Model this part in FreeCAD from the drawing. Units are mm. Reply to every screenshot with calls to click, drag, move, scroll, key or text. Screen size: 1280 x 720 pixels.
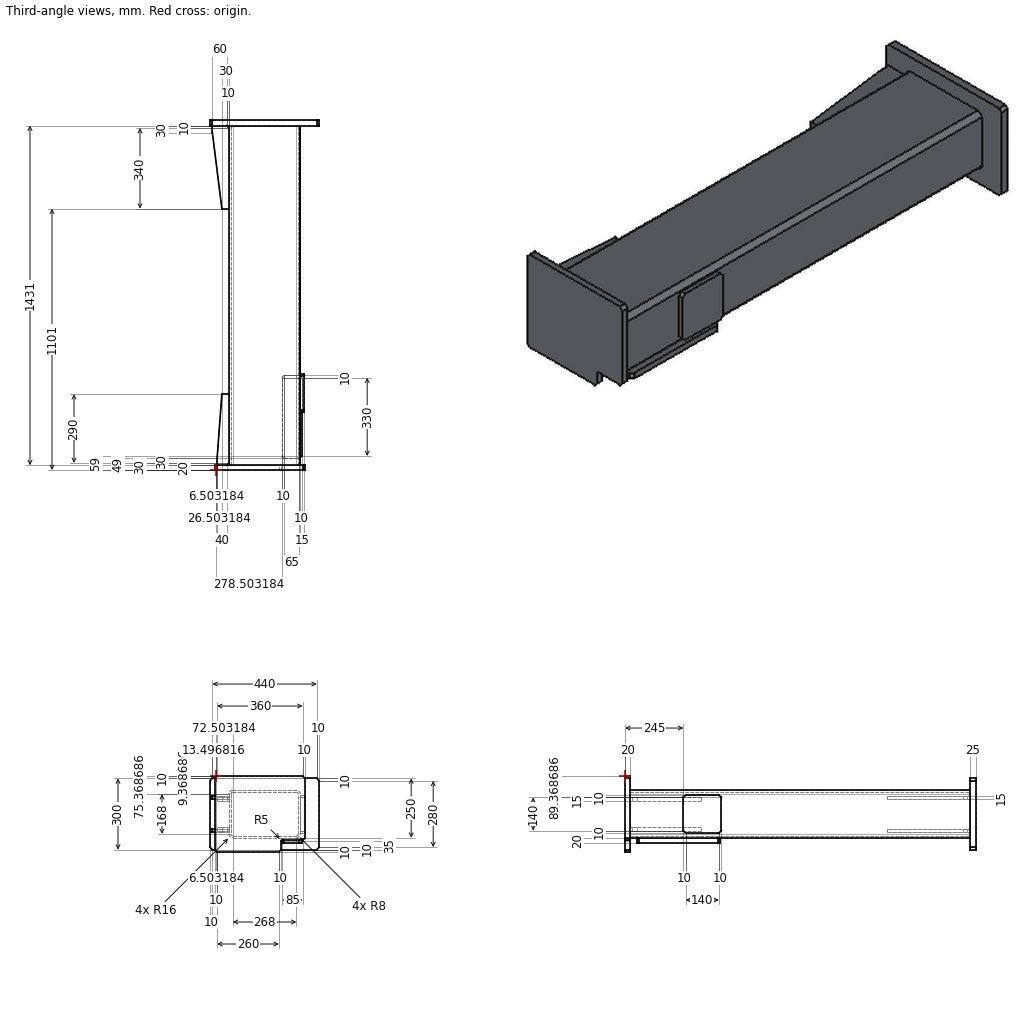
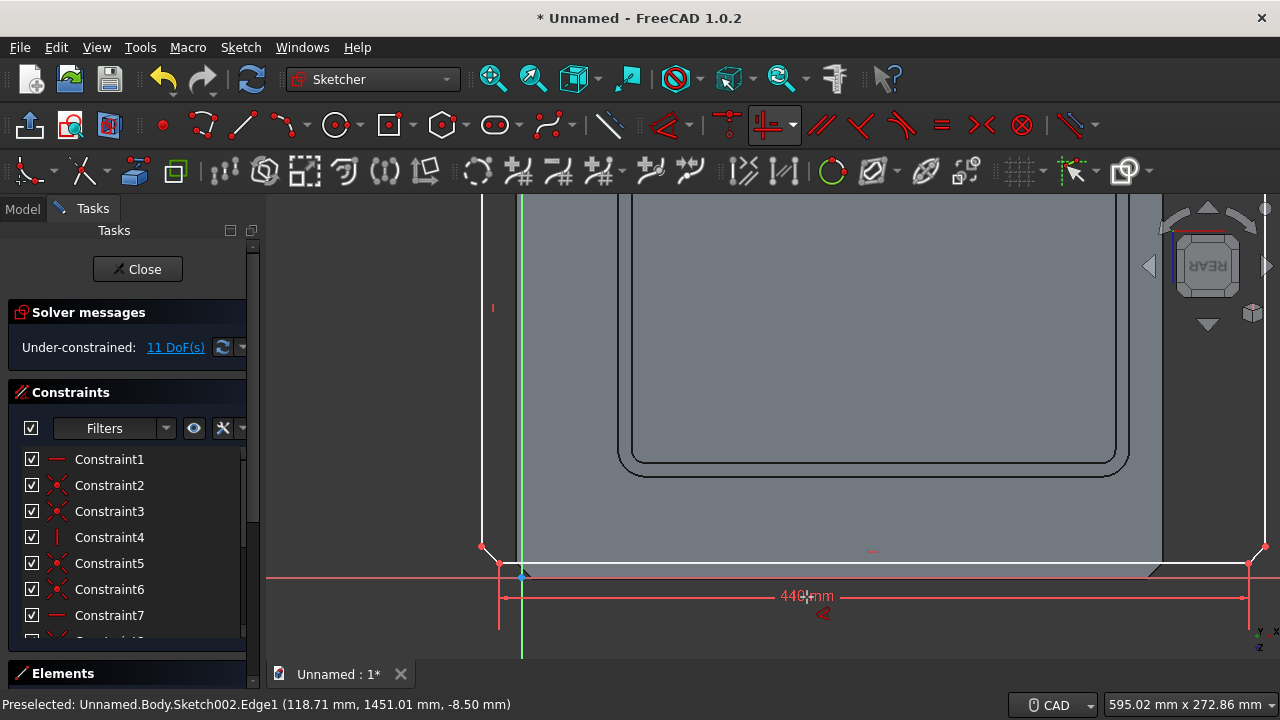
scroll(499, 563, down, 3)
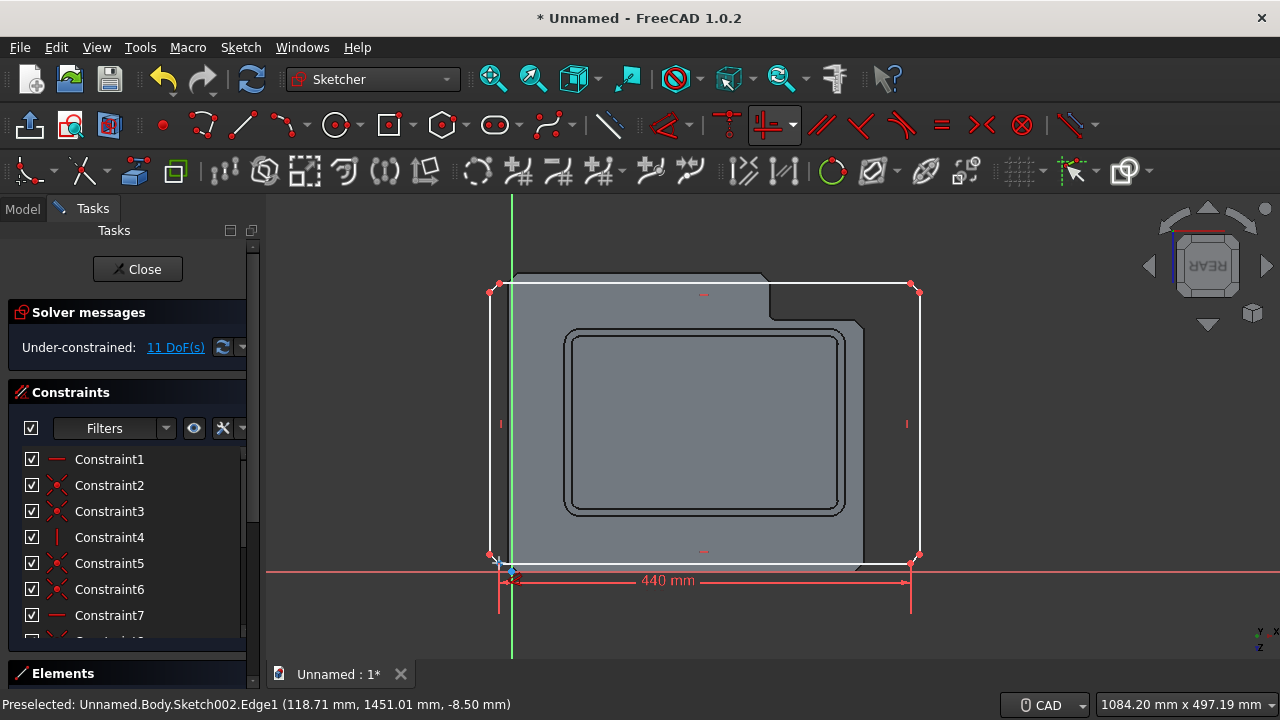
click(920, 476)
click(954, 423)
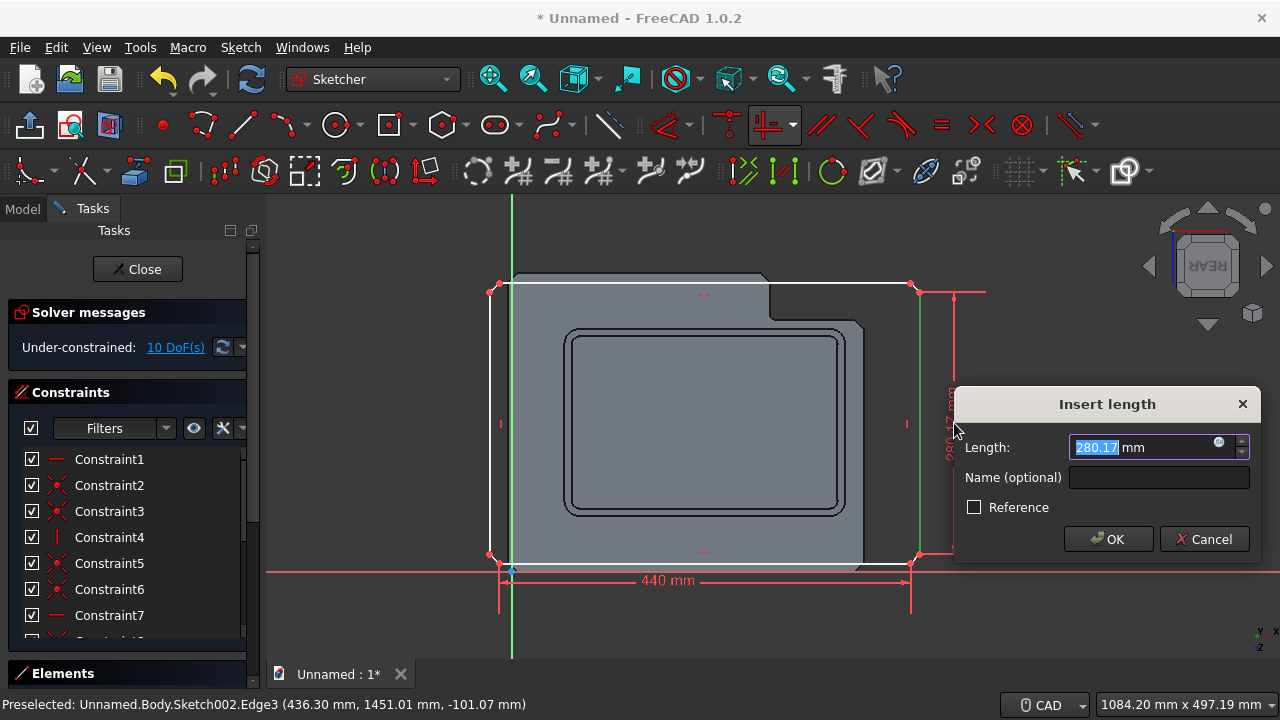
text(280)
key(Return)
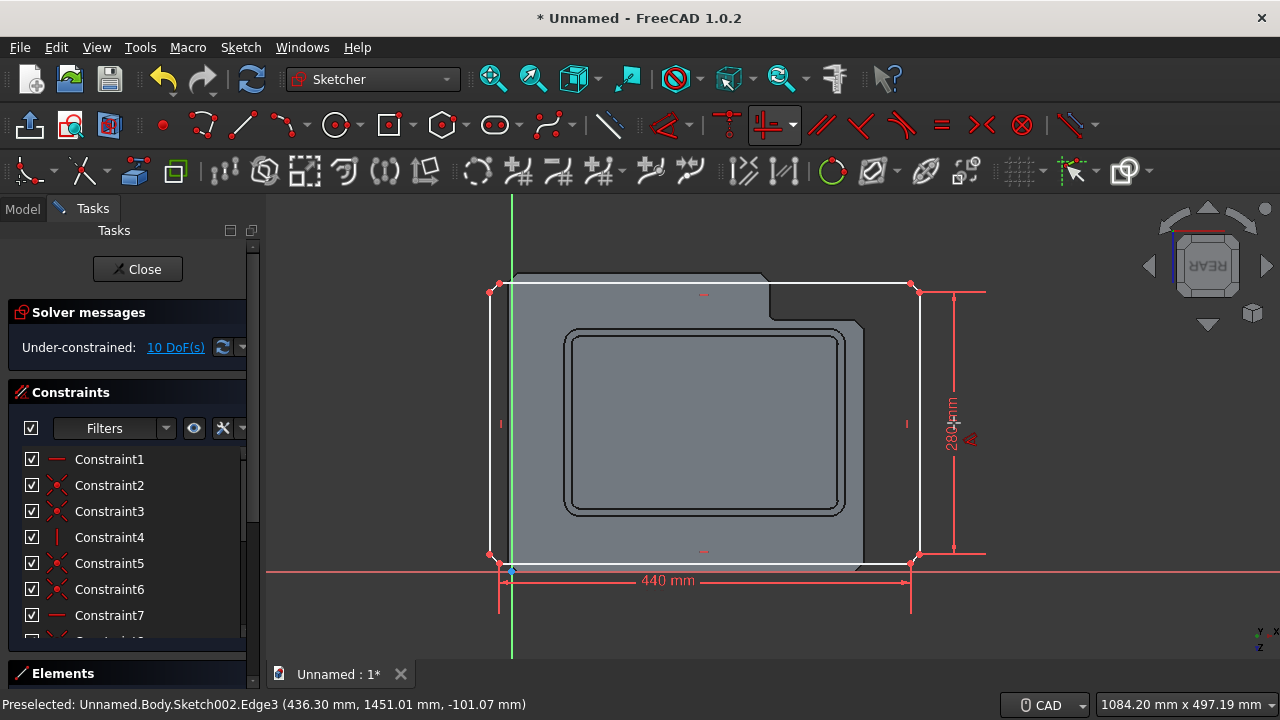
click(787, 283)
click(705, 249)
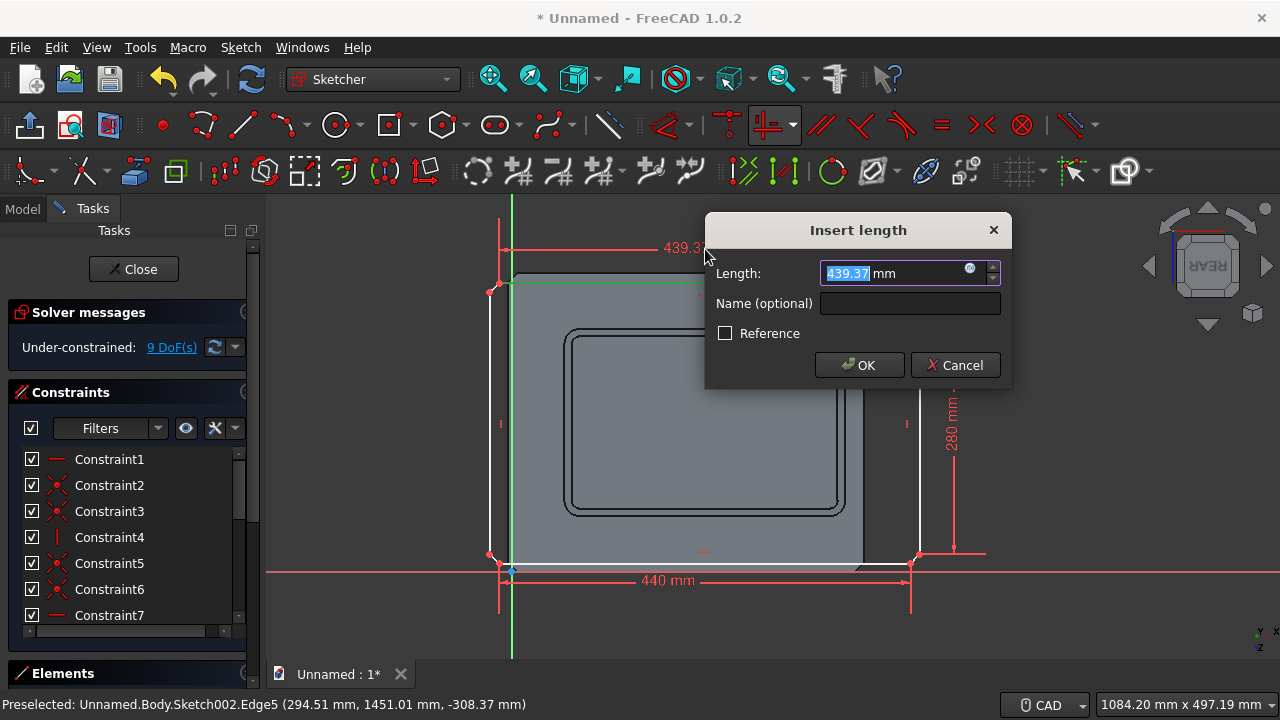
text(440)
key(Return)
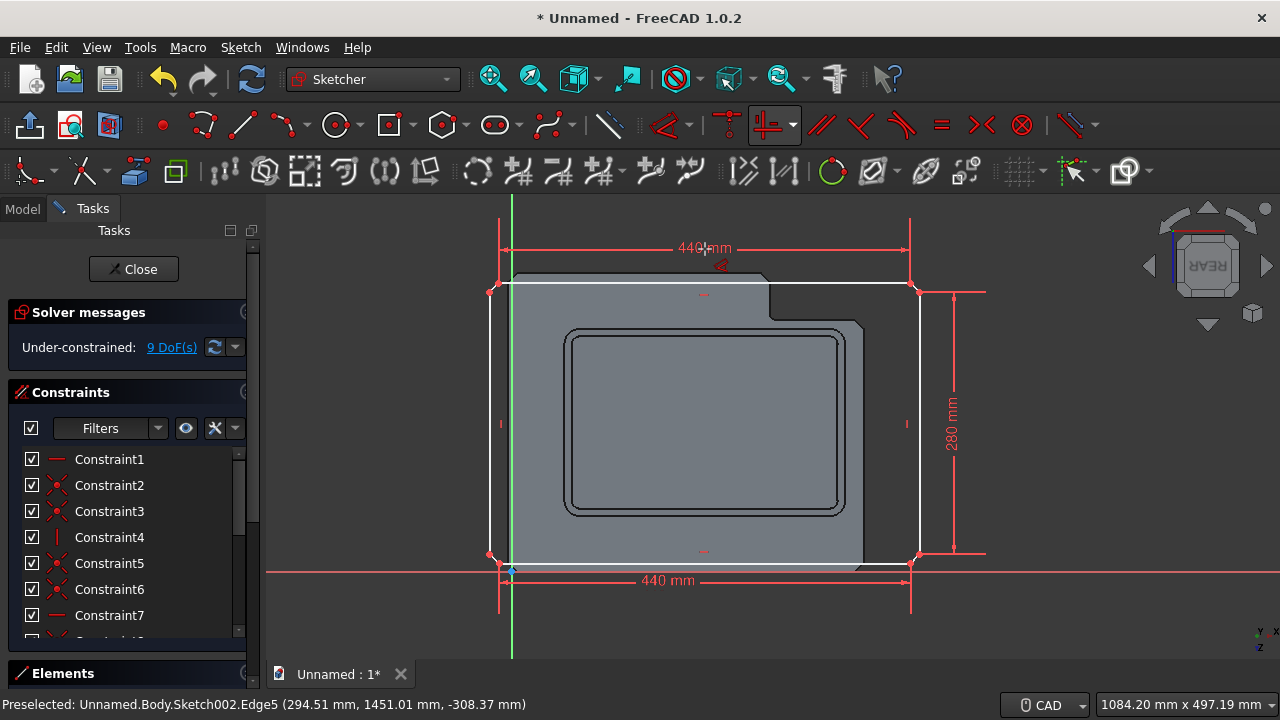
click(490, 371)
click(456, 423)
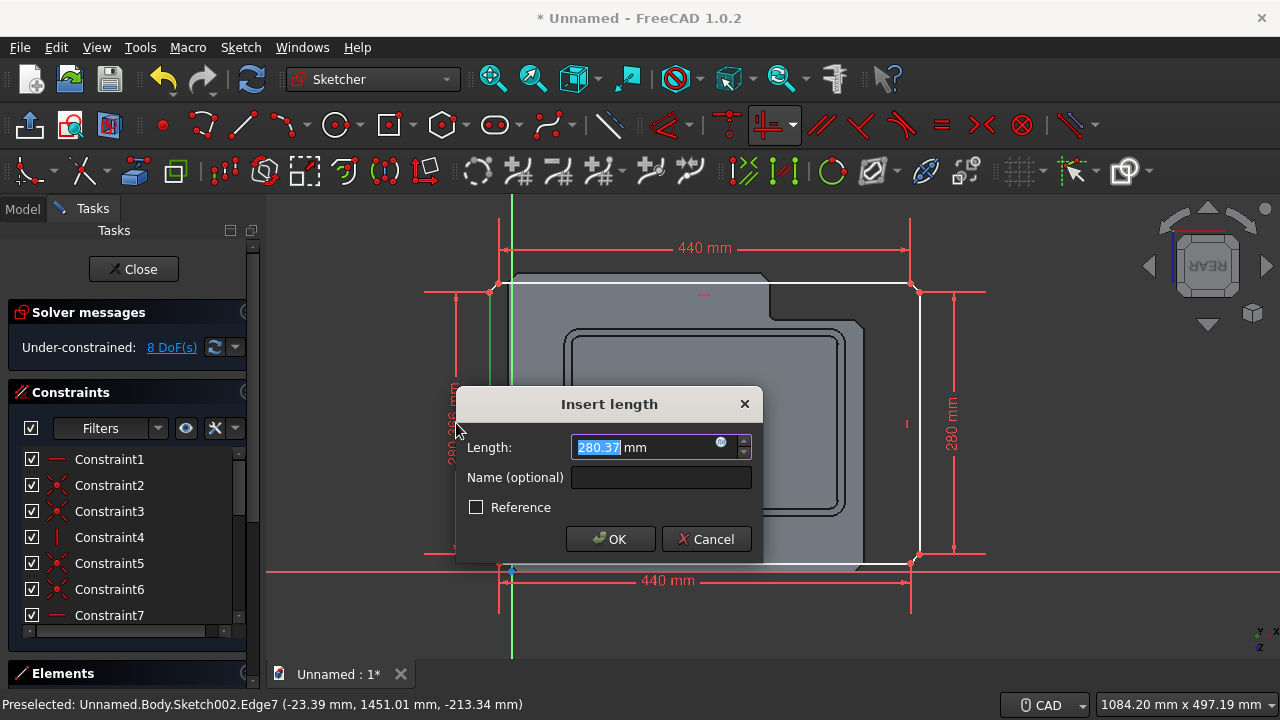
text(280)
key(Return)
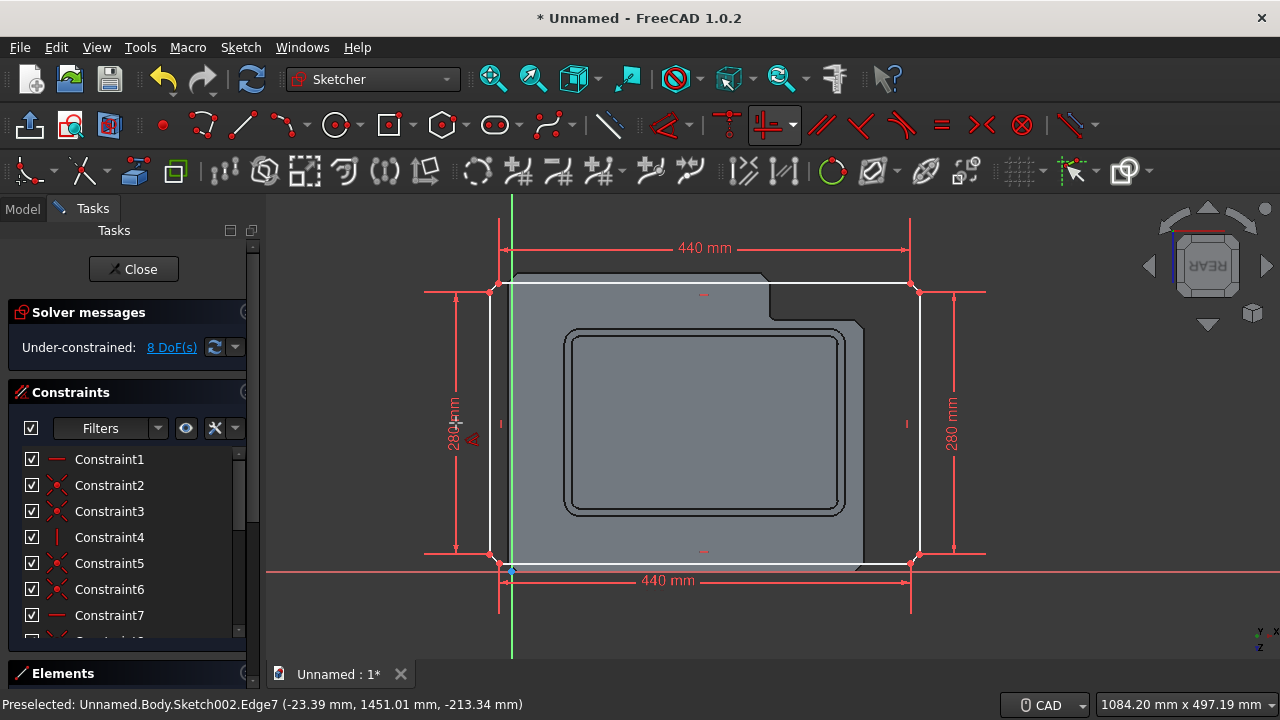
scroll(915, 559, up, 8)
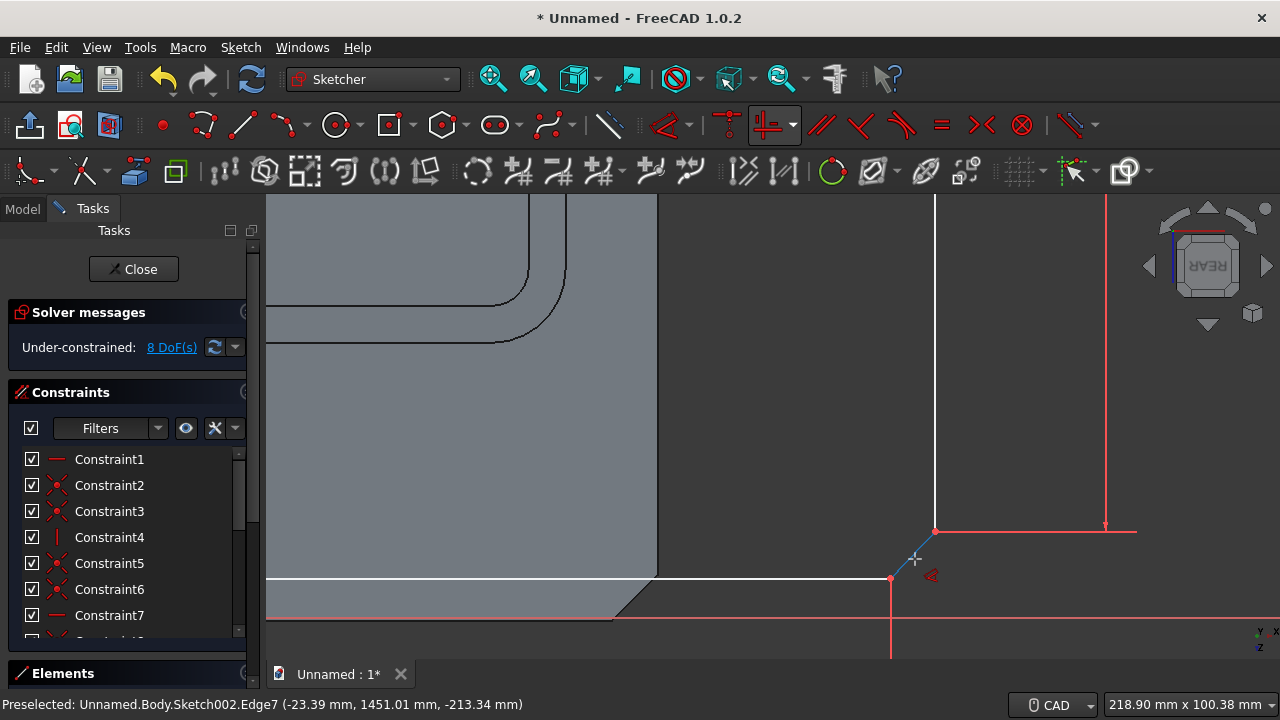
click(913, 555)
click(913, 498)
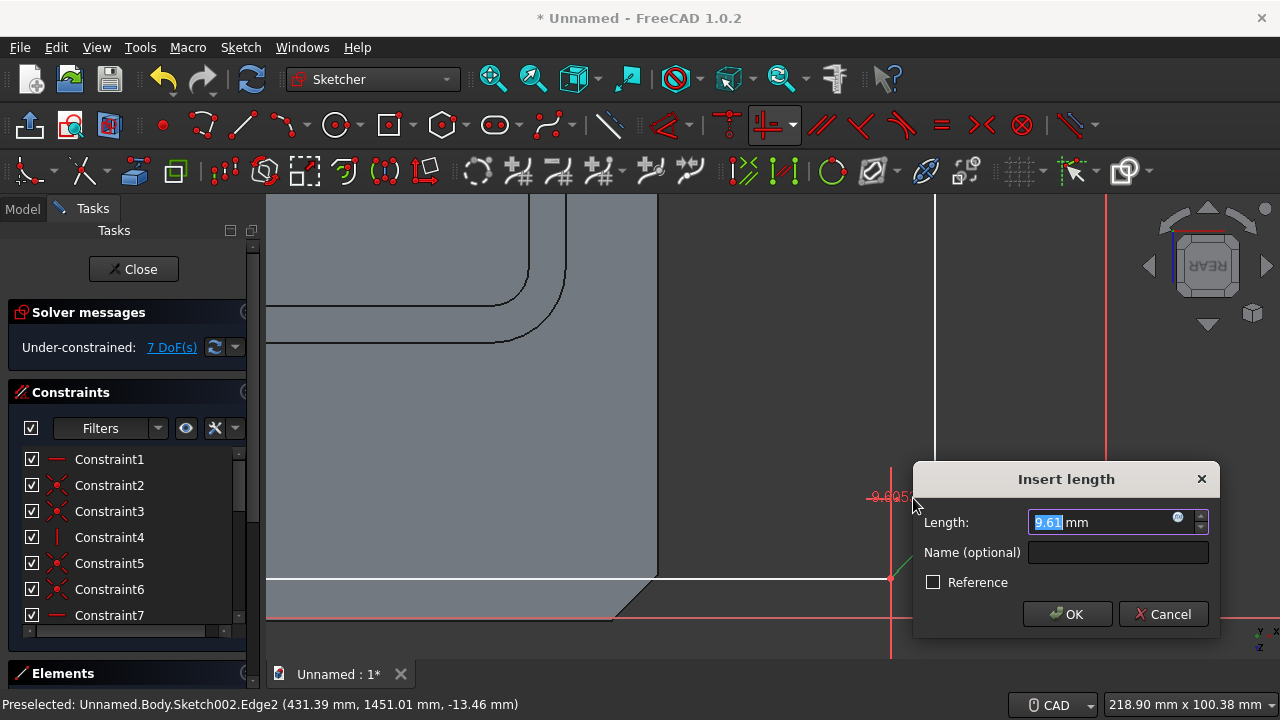
text(10)
key(Return)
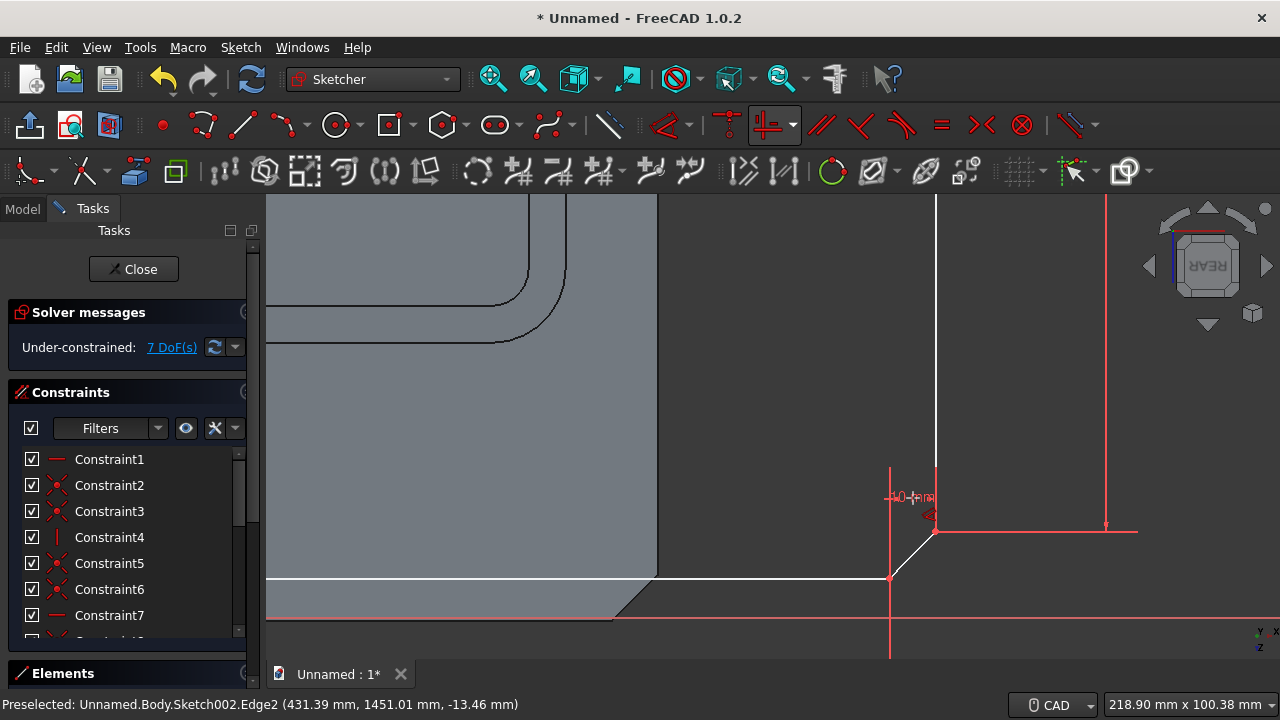
click(903, 564)
click(970, 555)